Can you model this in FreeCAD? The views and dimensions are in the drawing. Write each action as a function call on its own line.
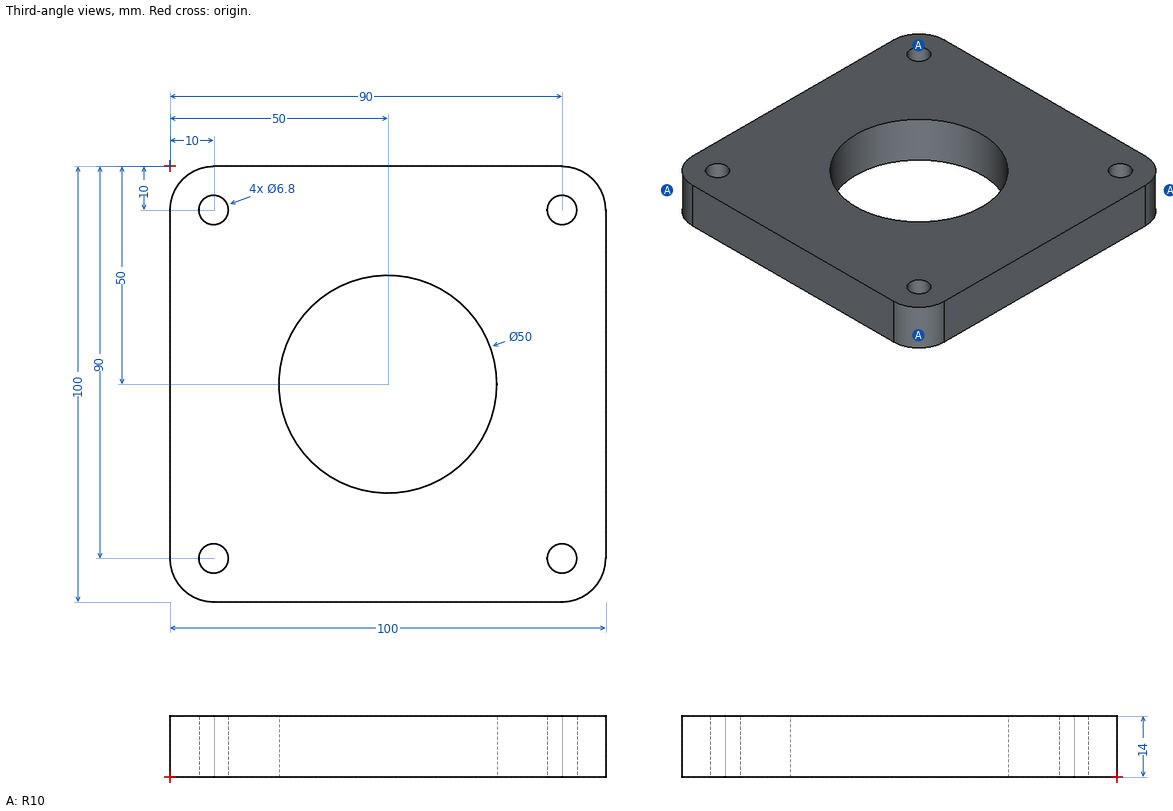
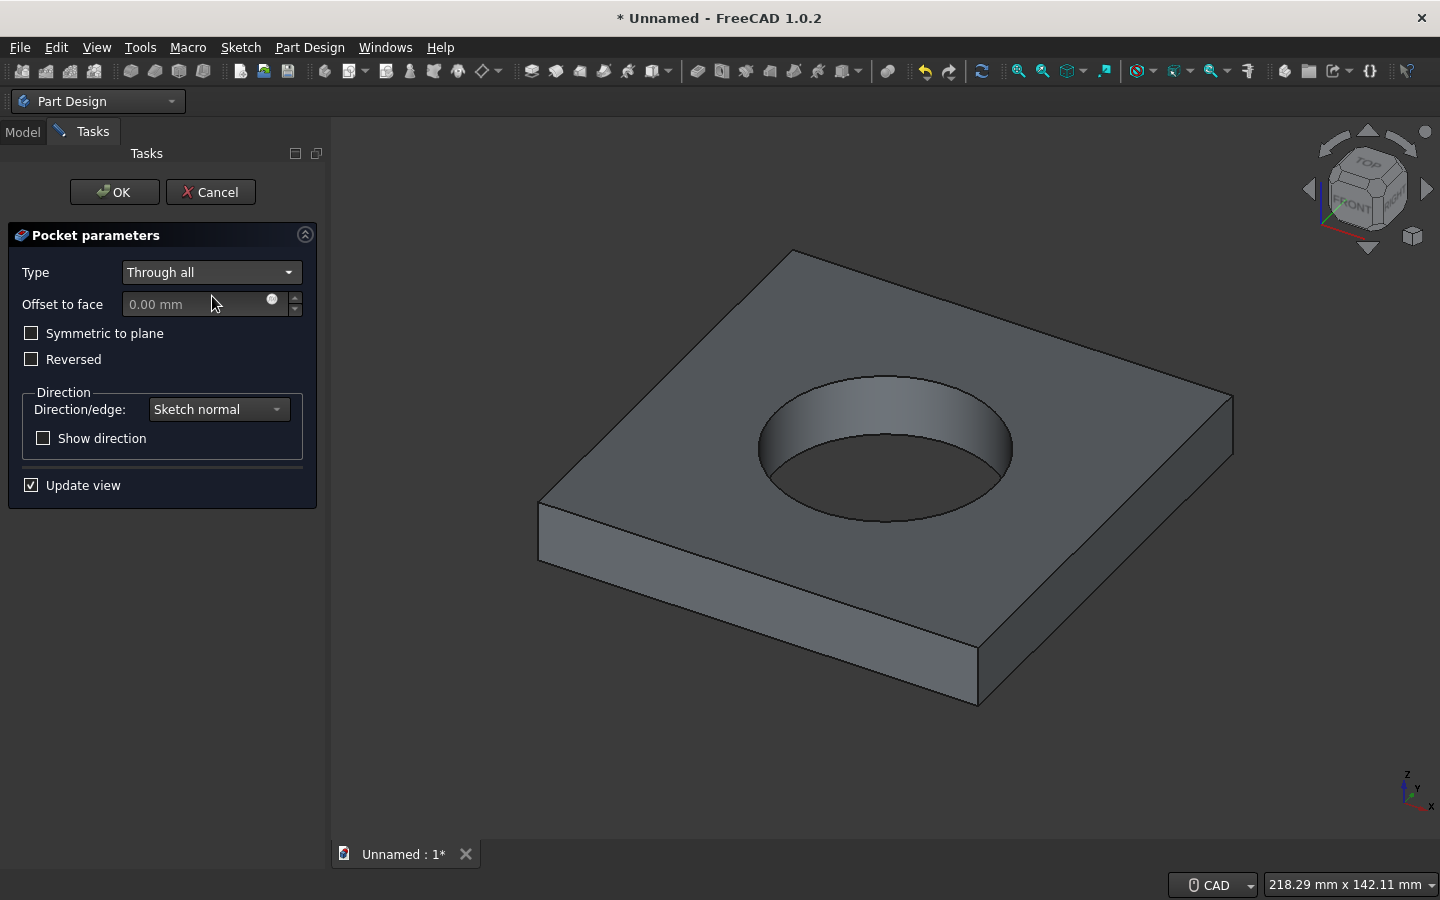
click(115, 192)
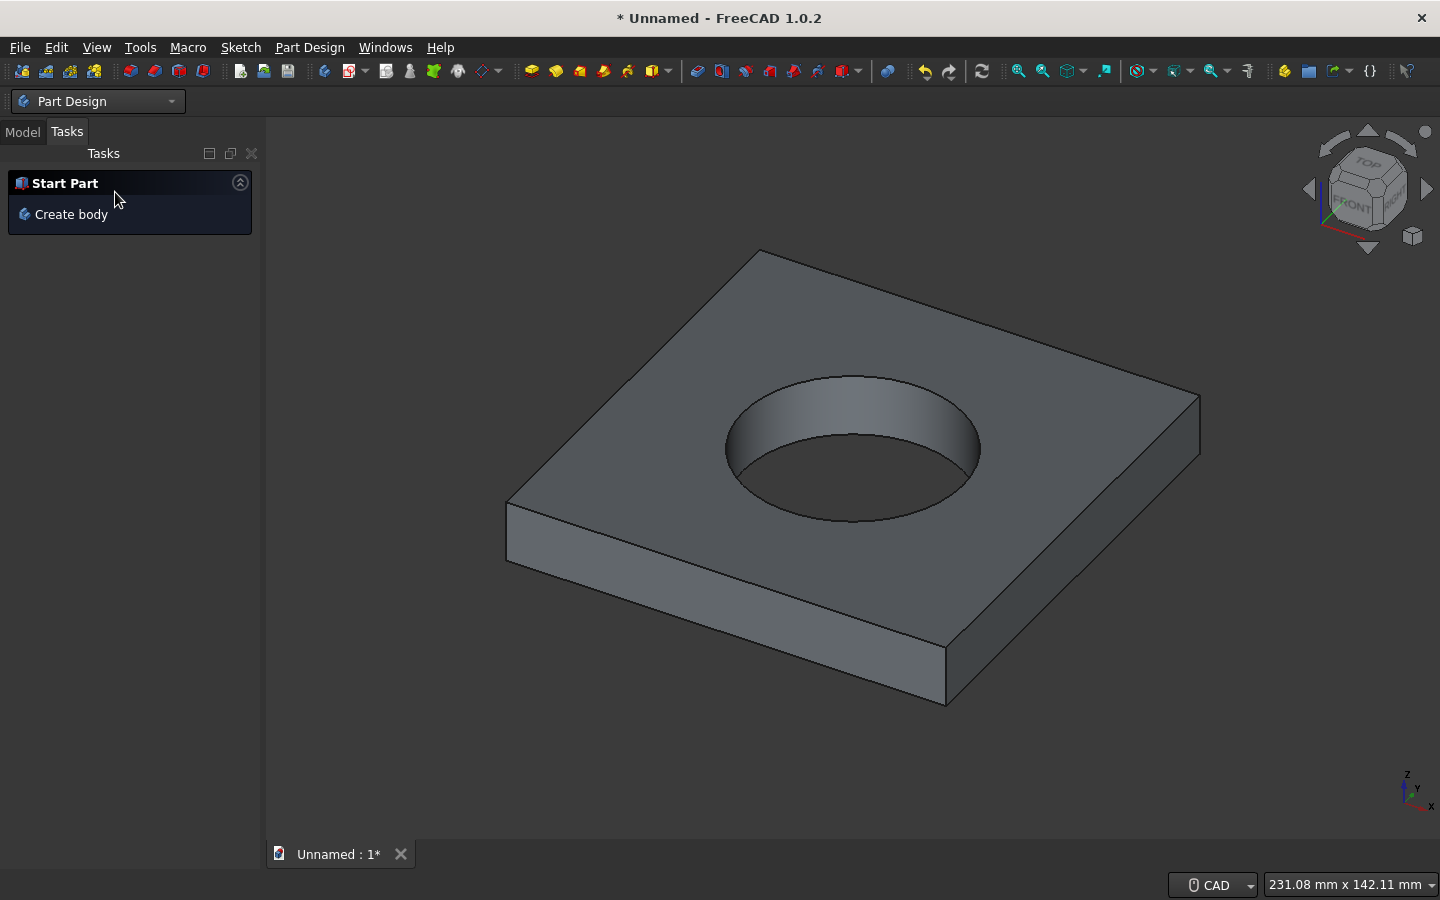
click(800, 334)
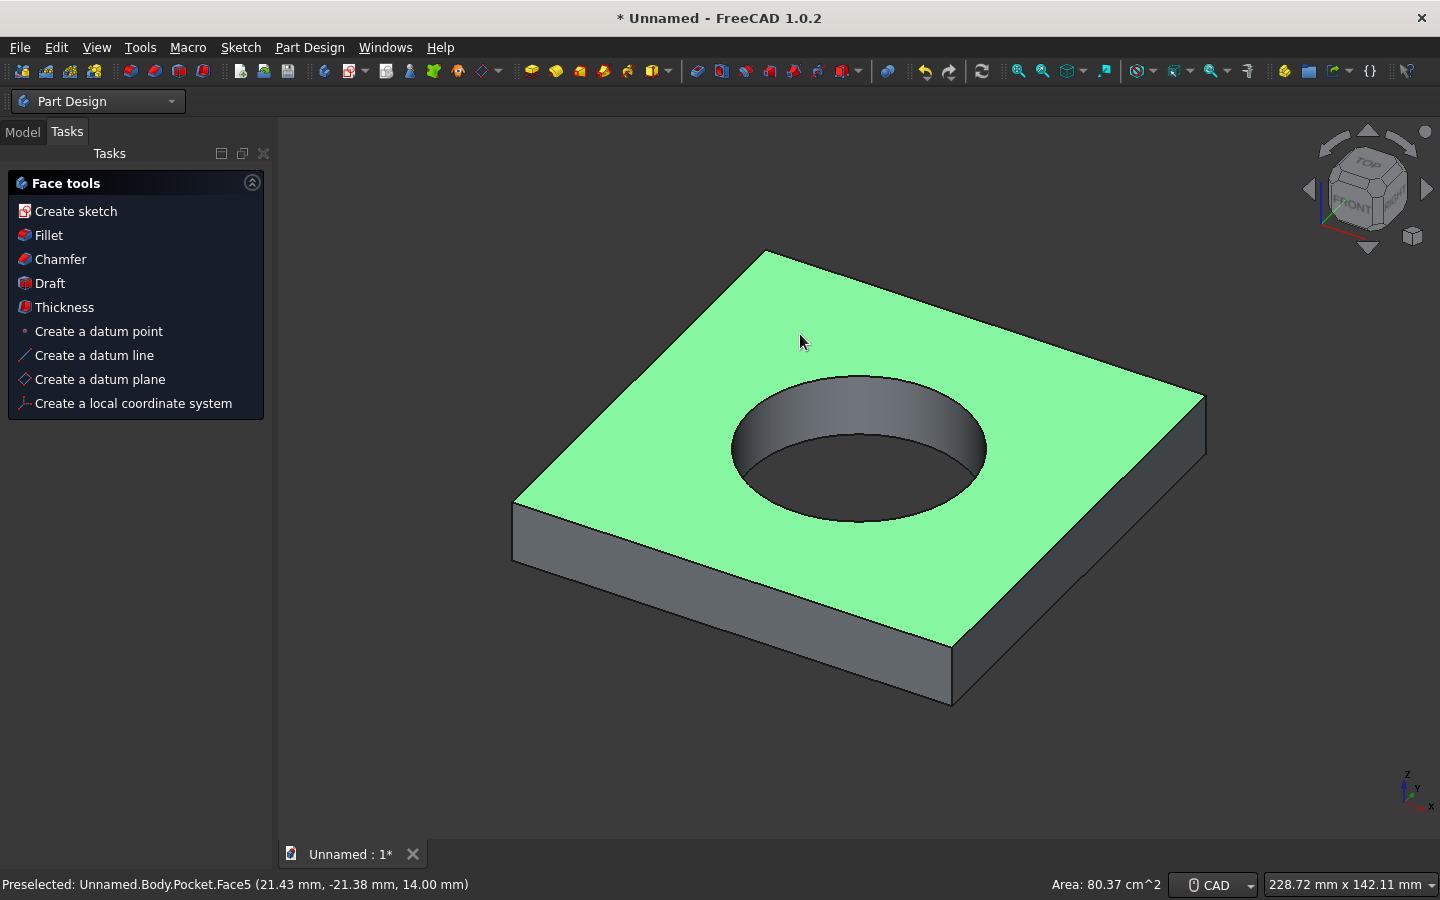
click(350, 72)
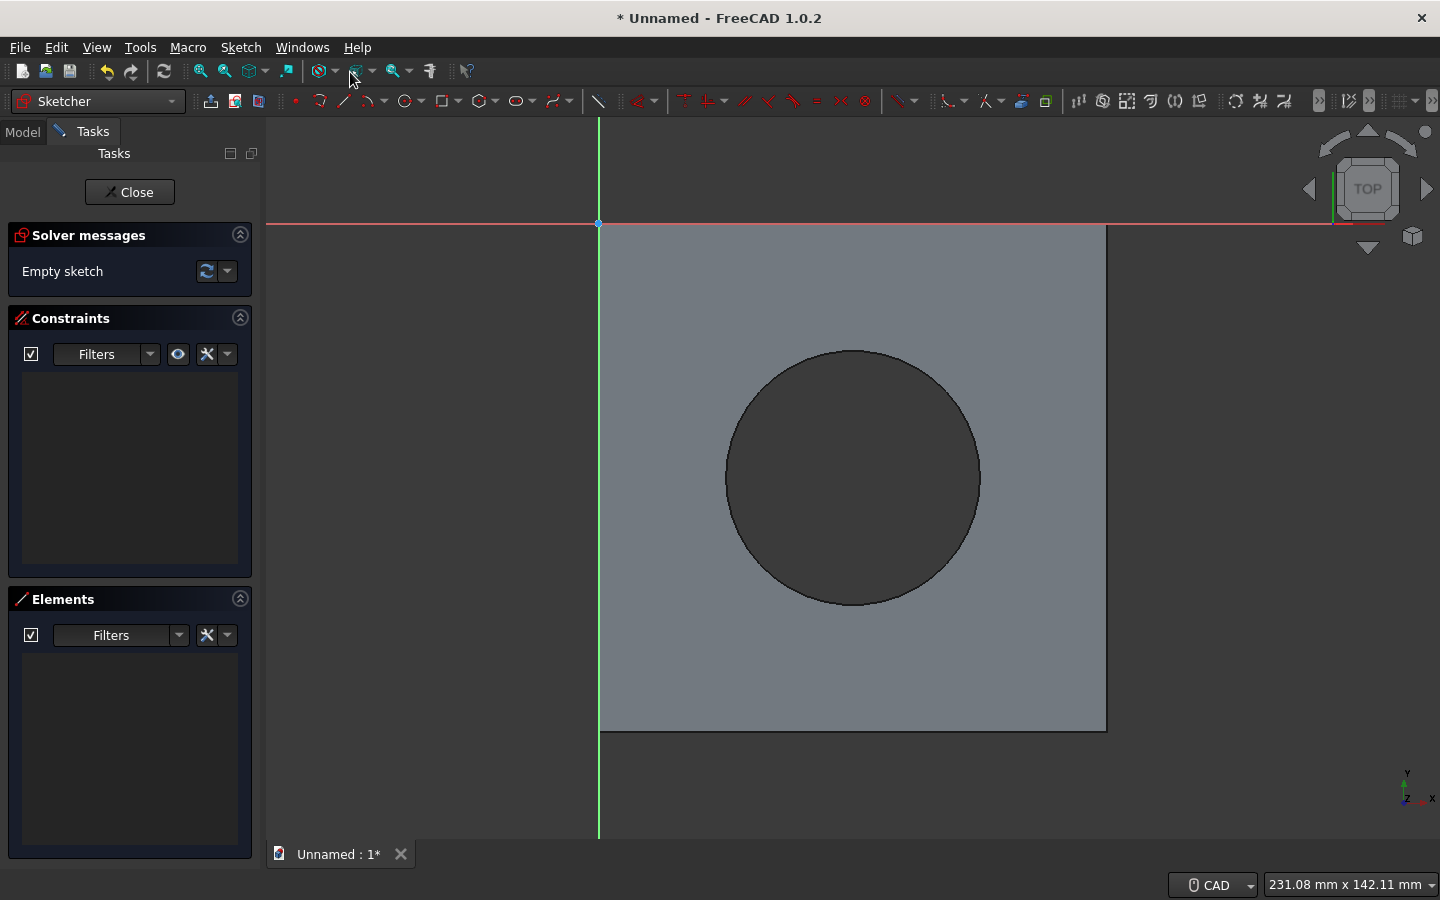
click(406, 102)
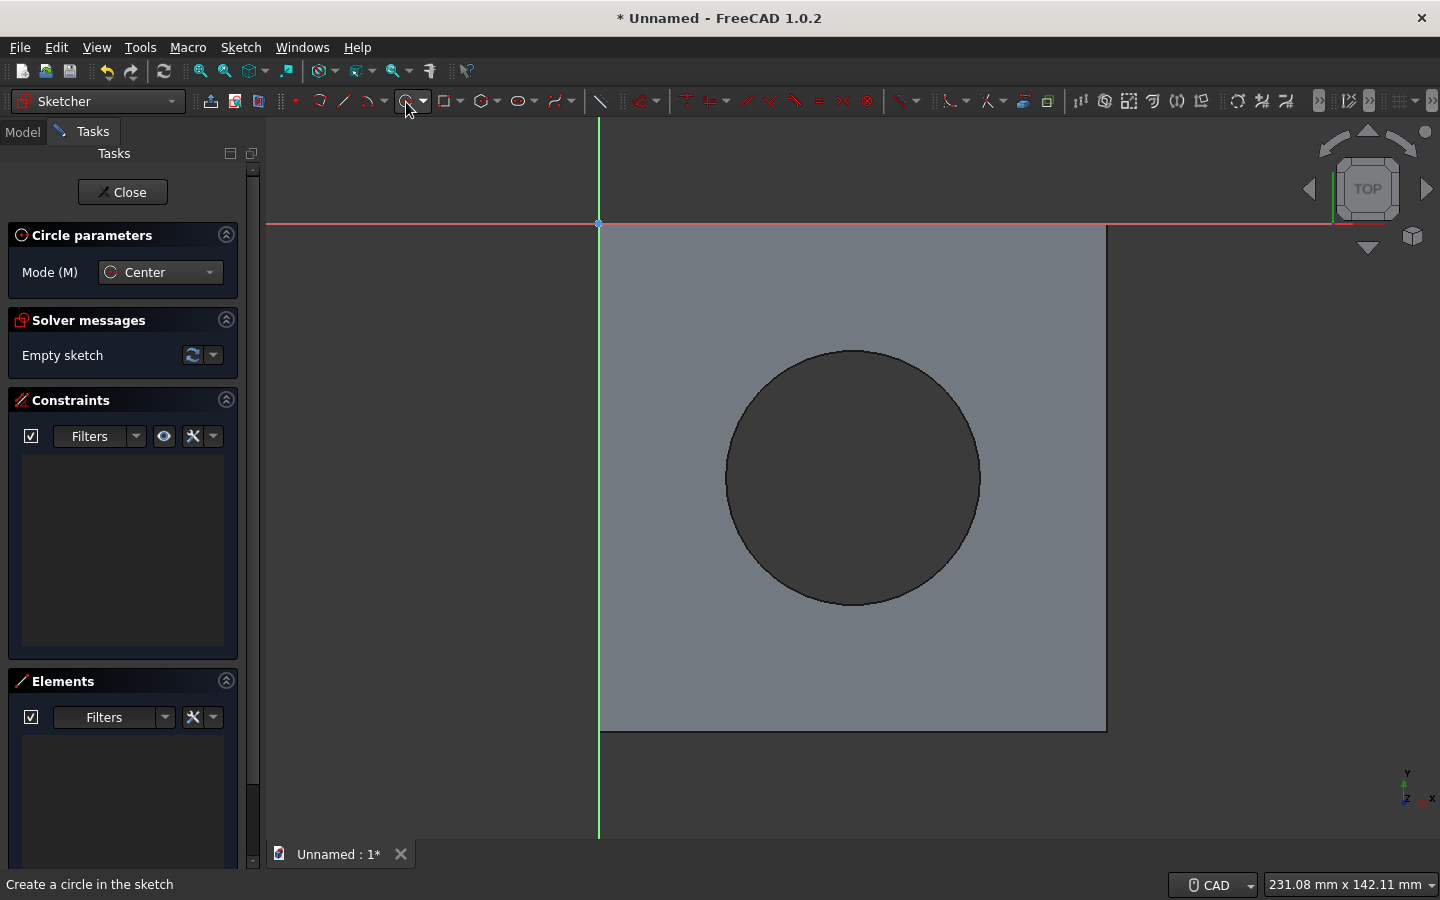
scroll(650, 275, up, 2)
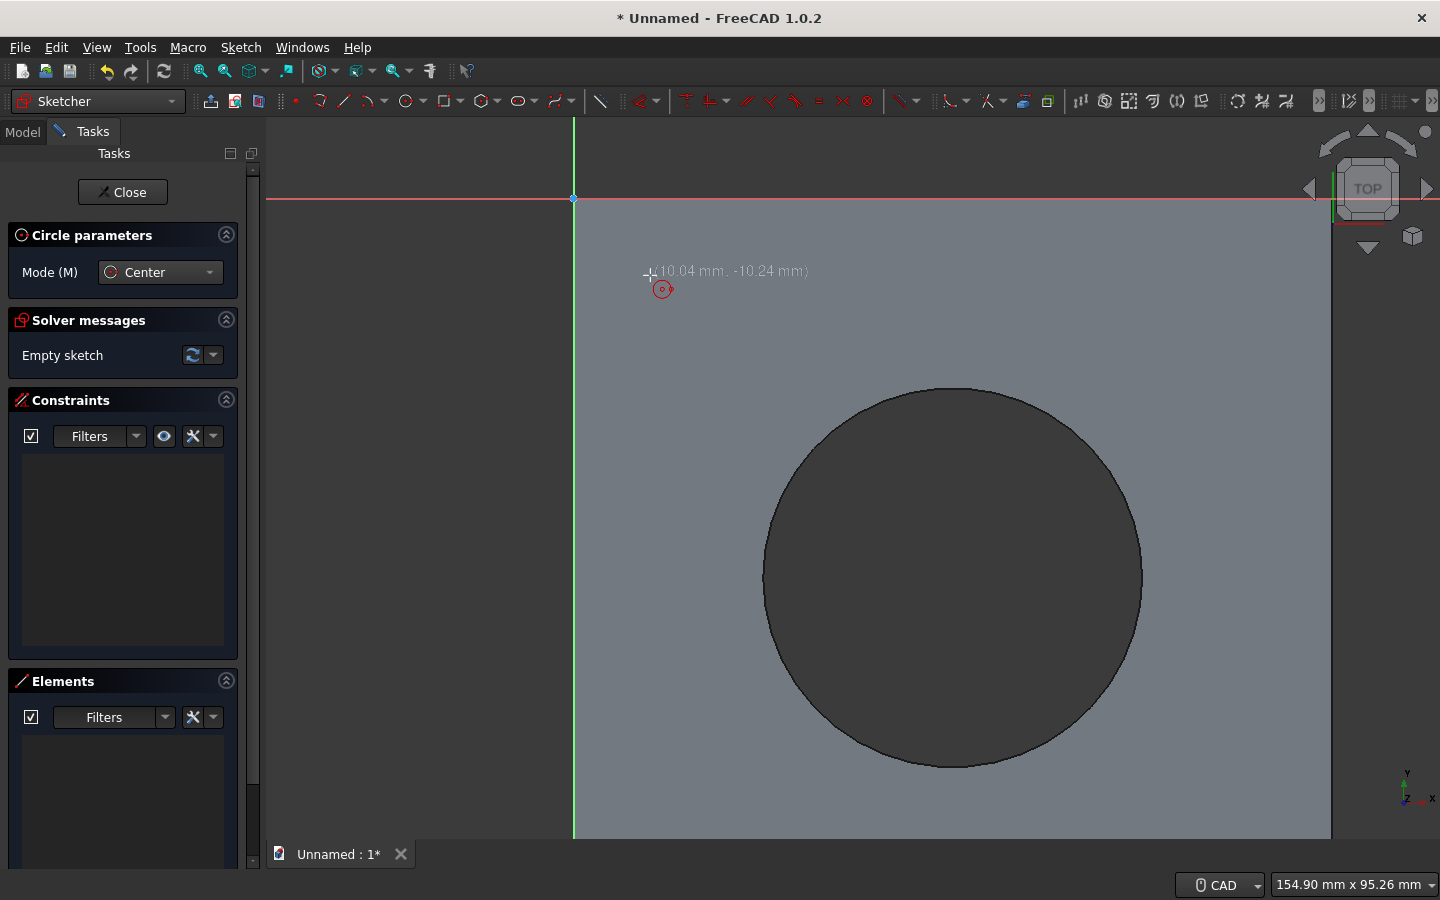
click(650, 275)
click(668, 256)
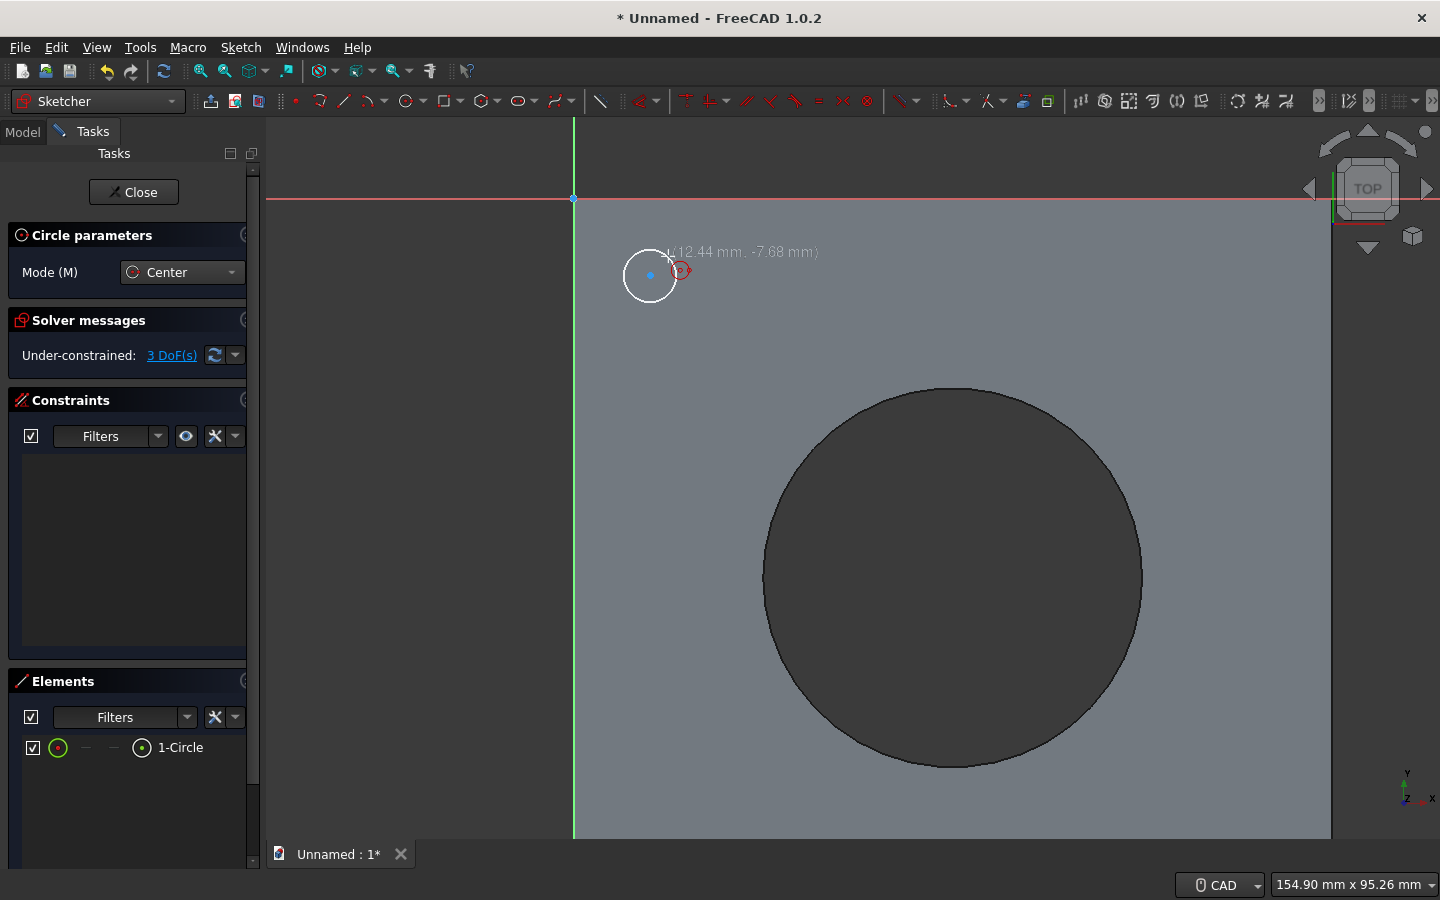
click(1256, 275)
click(1274, 256)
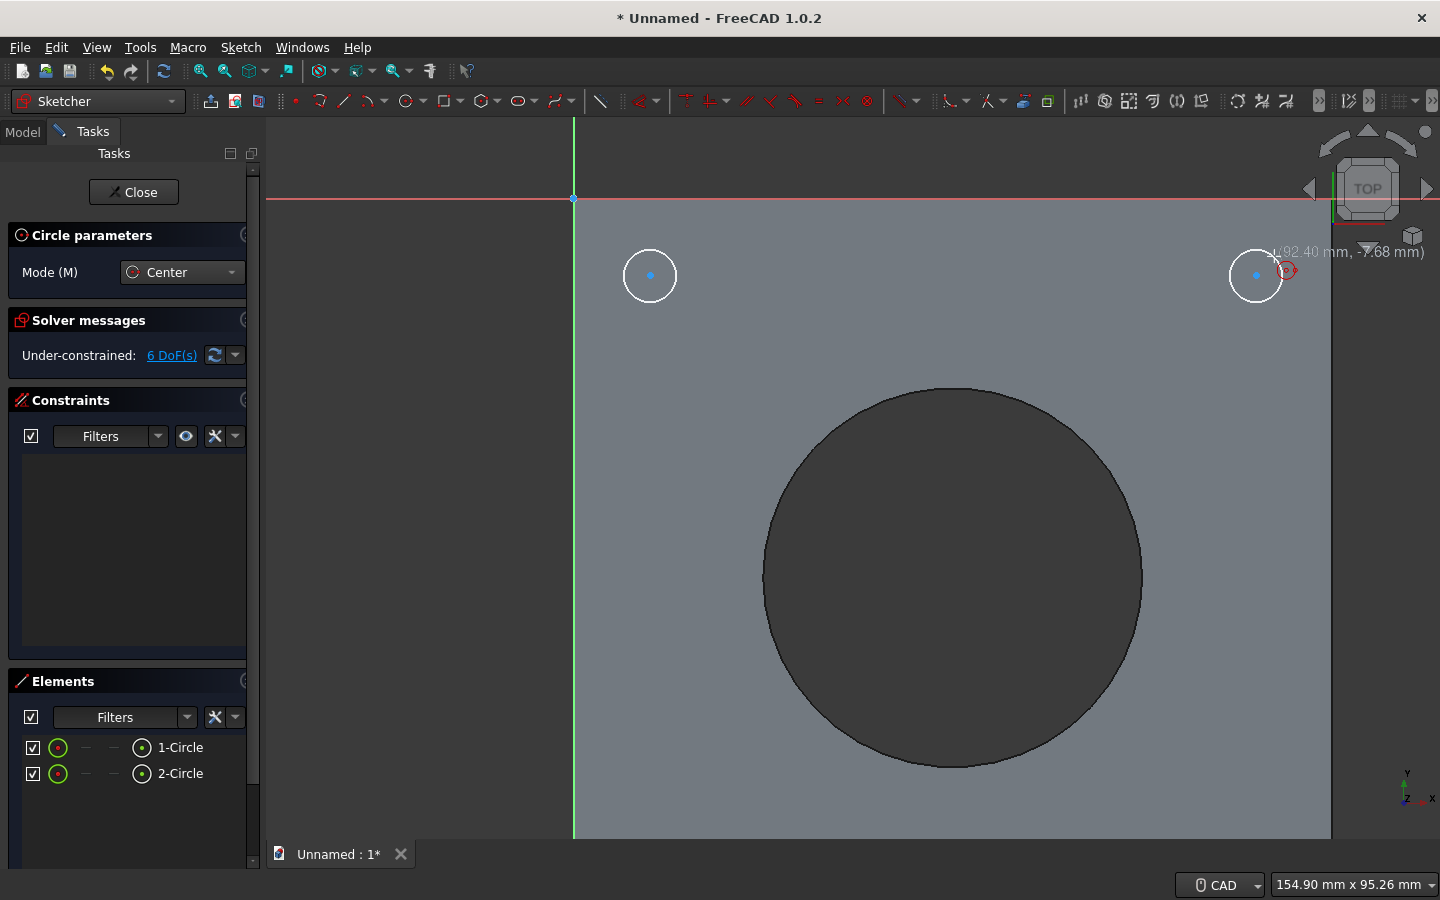
scroll(493, 326, down, 2)